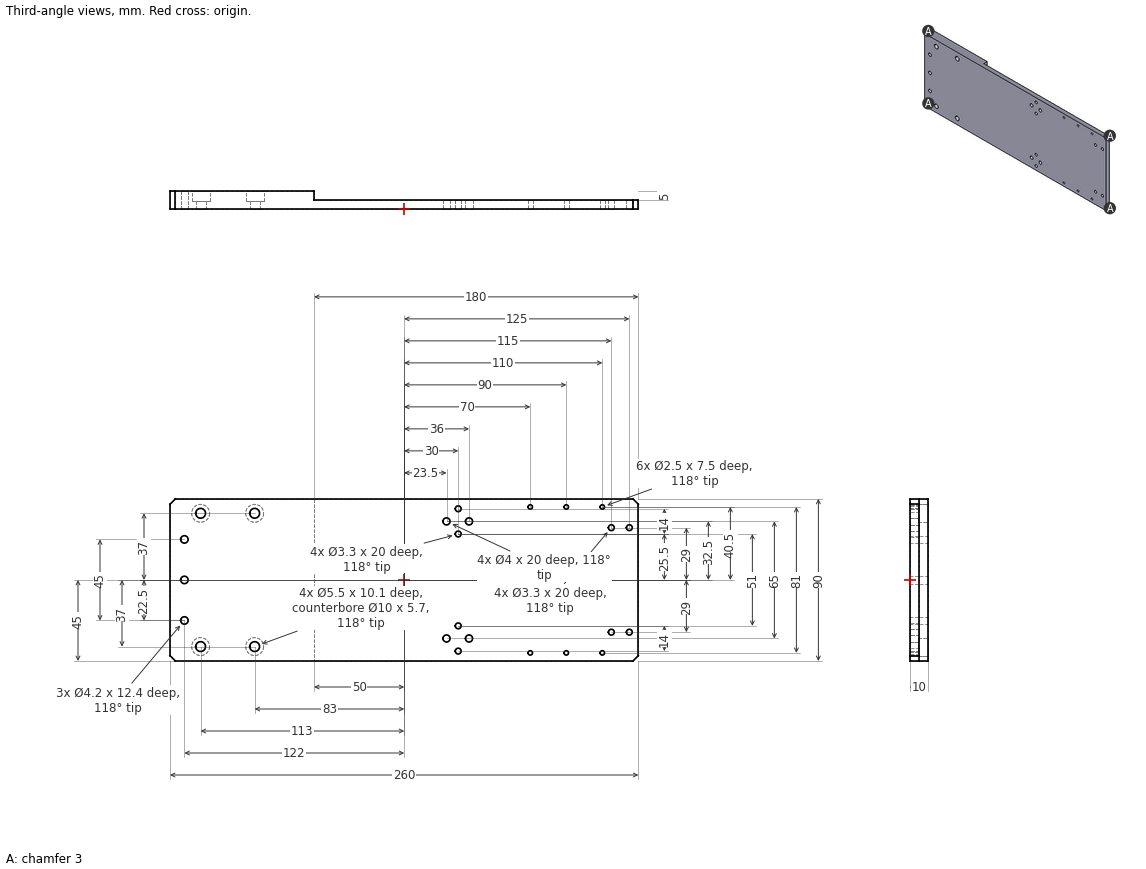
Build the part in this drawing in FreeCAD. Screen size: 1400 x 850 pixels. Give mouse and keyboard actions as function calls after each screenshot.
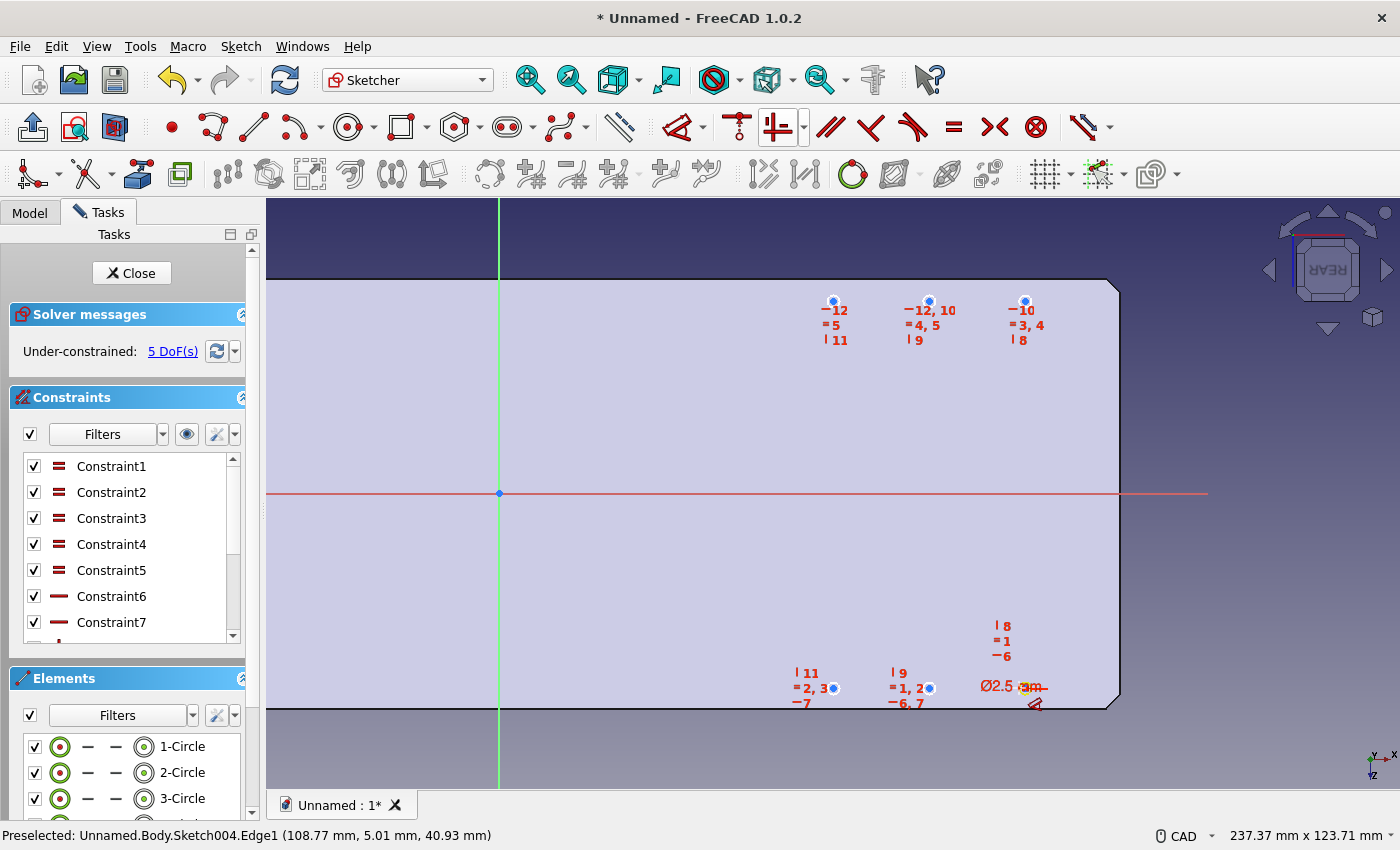
click(929, 689)
click(714, 723)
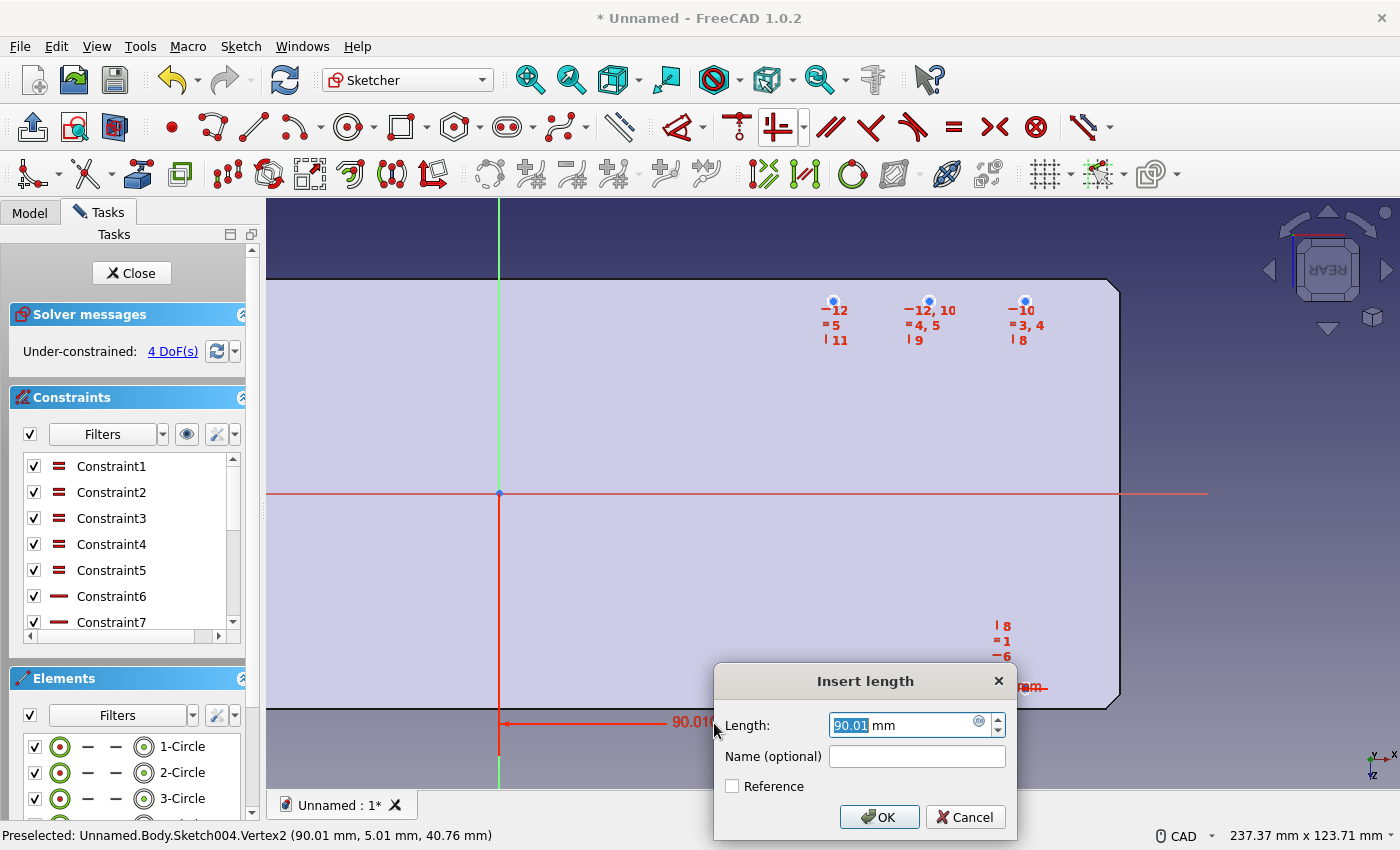
text(90)
key(Return)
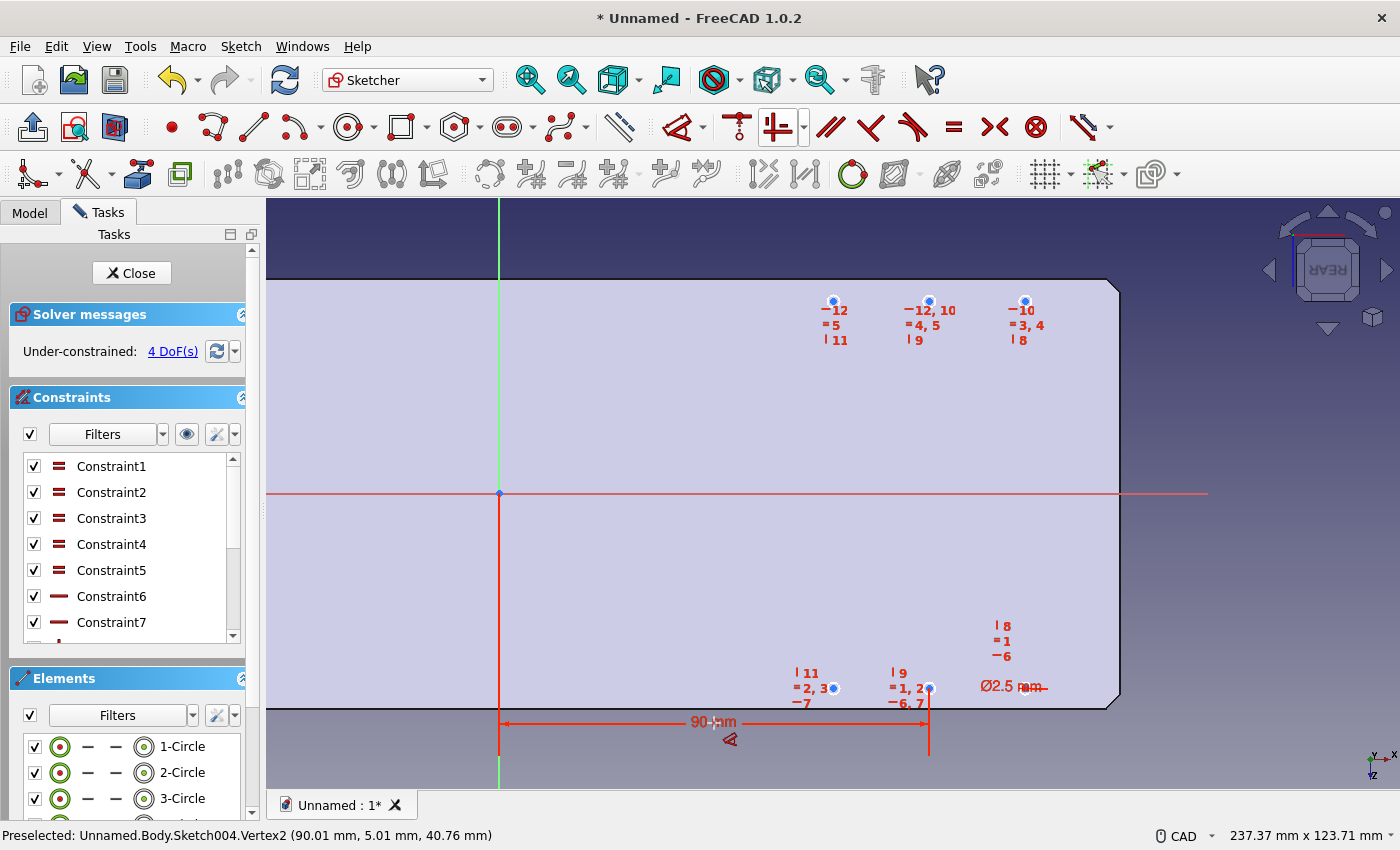
click(834, 689)
click(590, 723)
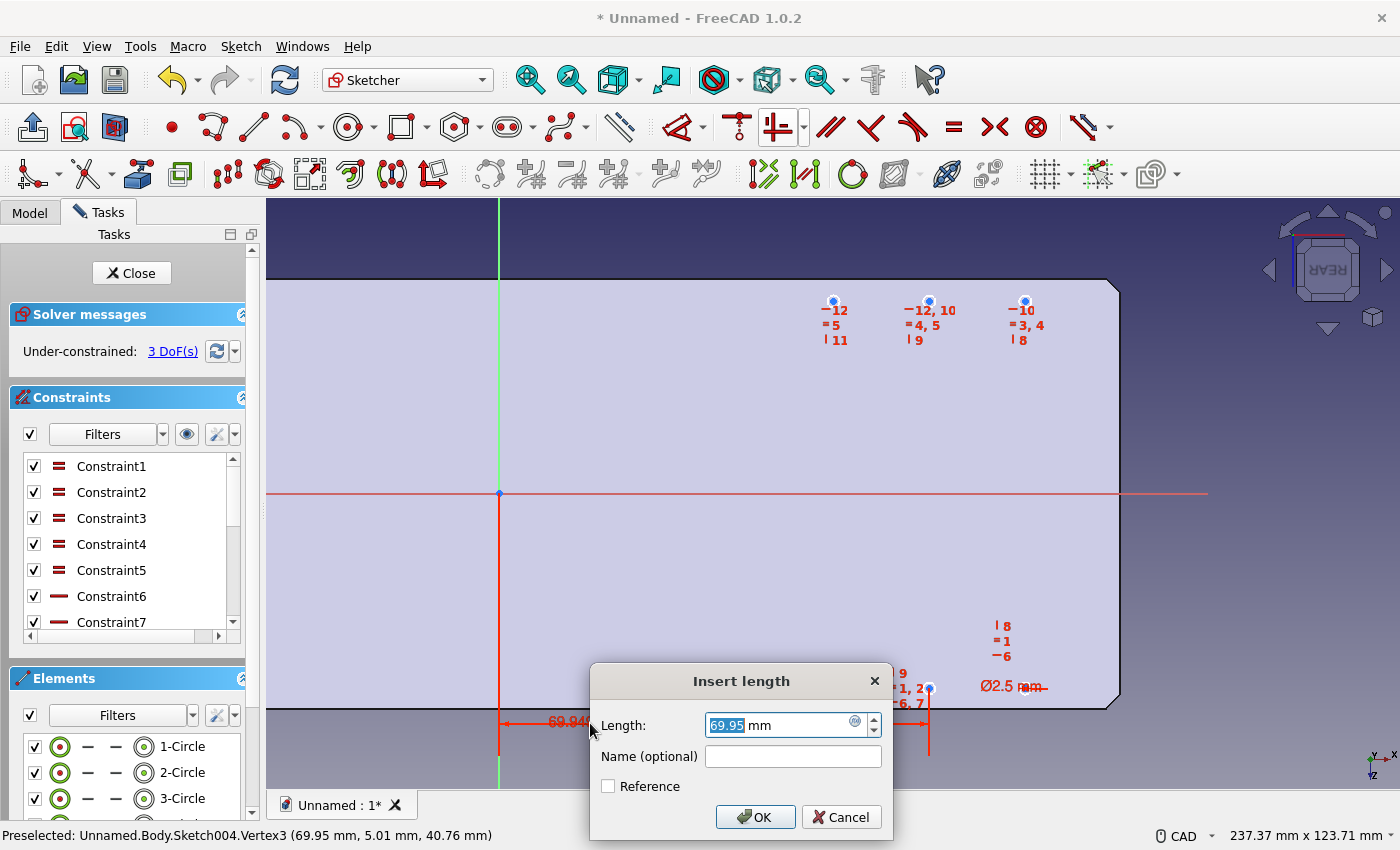
text(70)
key(Return)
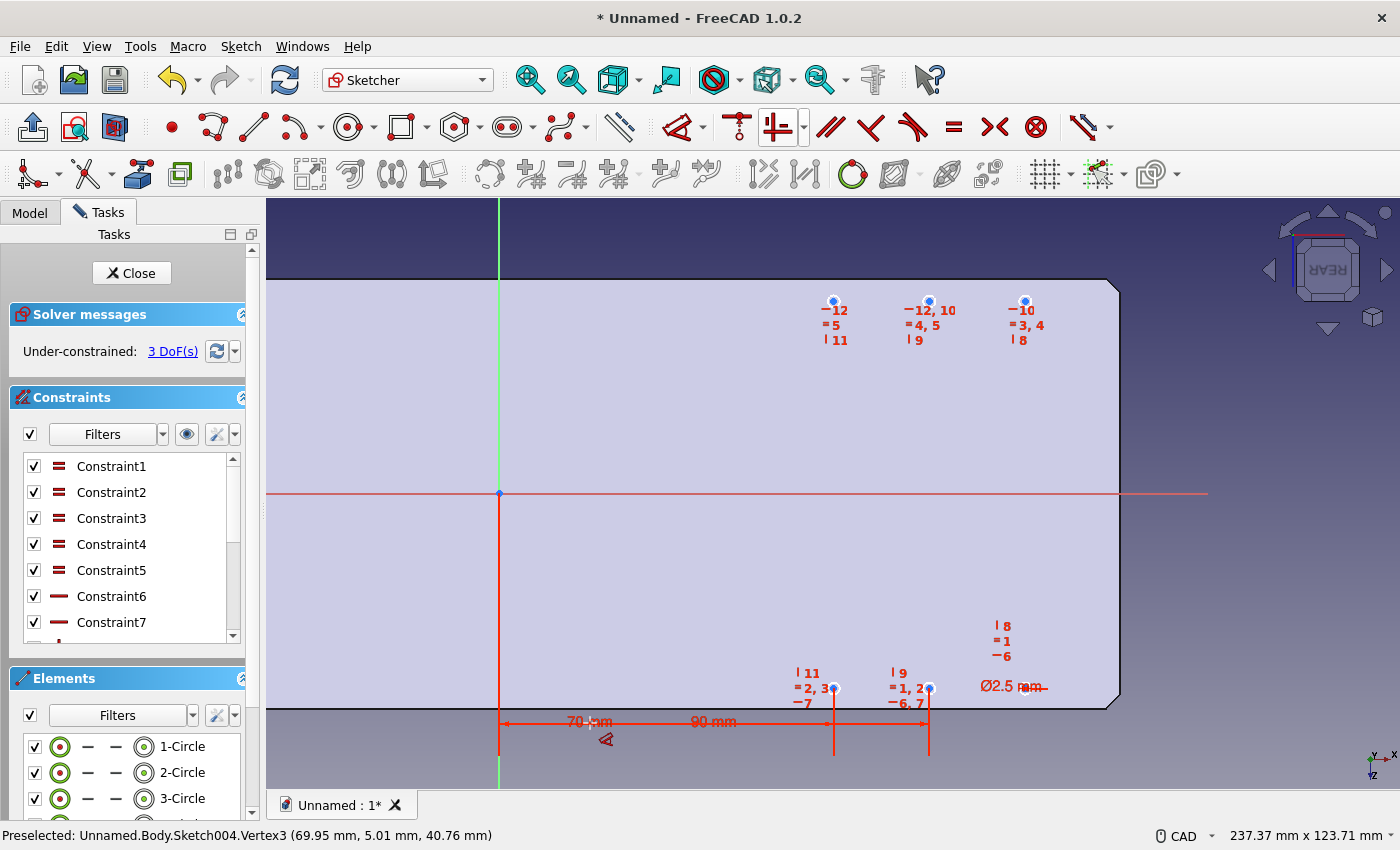
click(1025, 689)
click(883, 723)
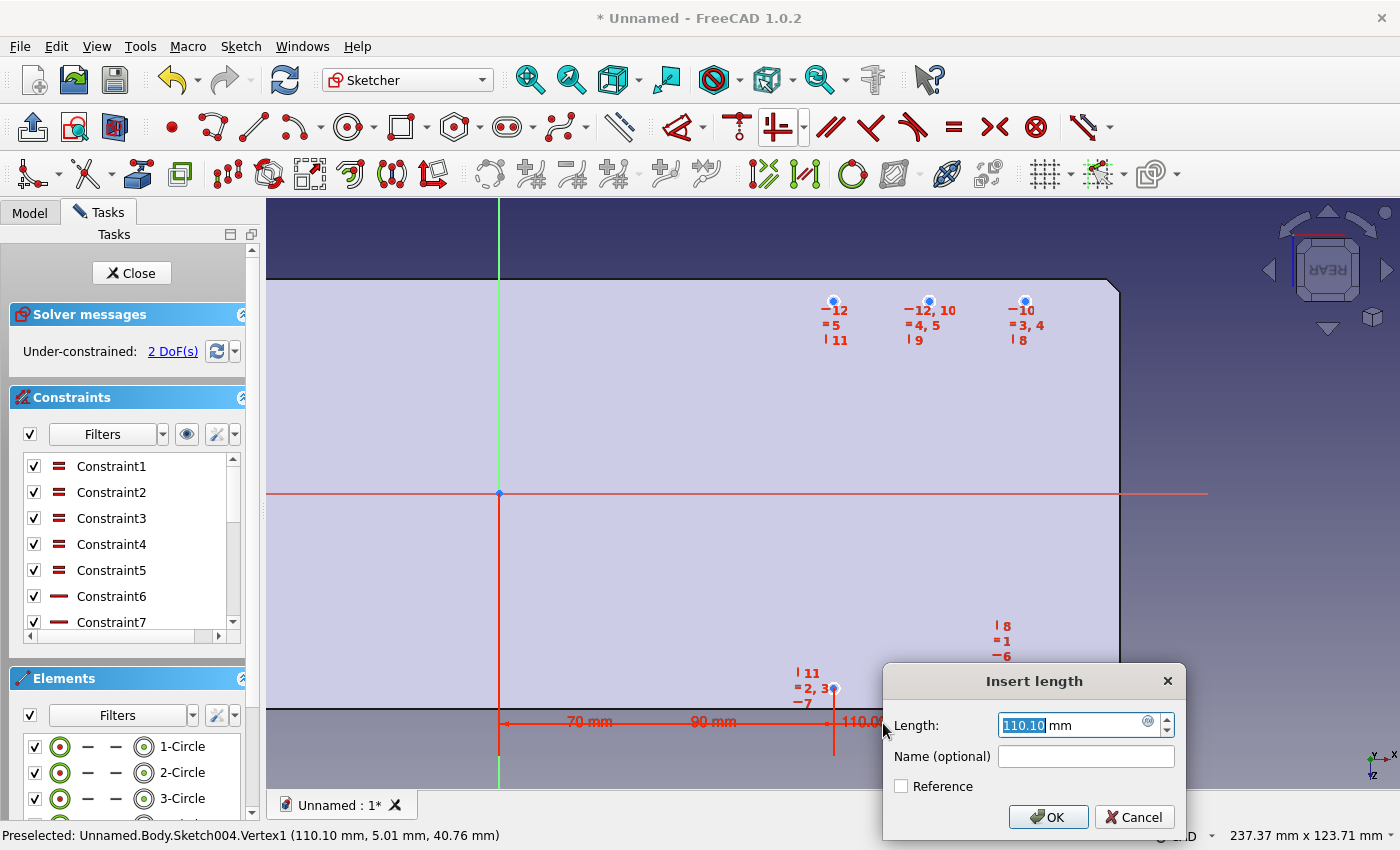
text(110)
key(Return)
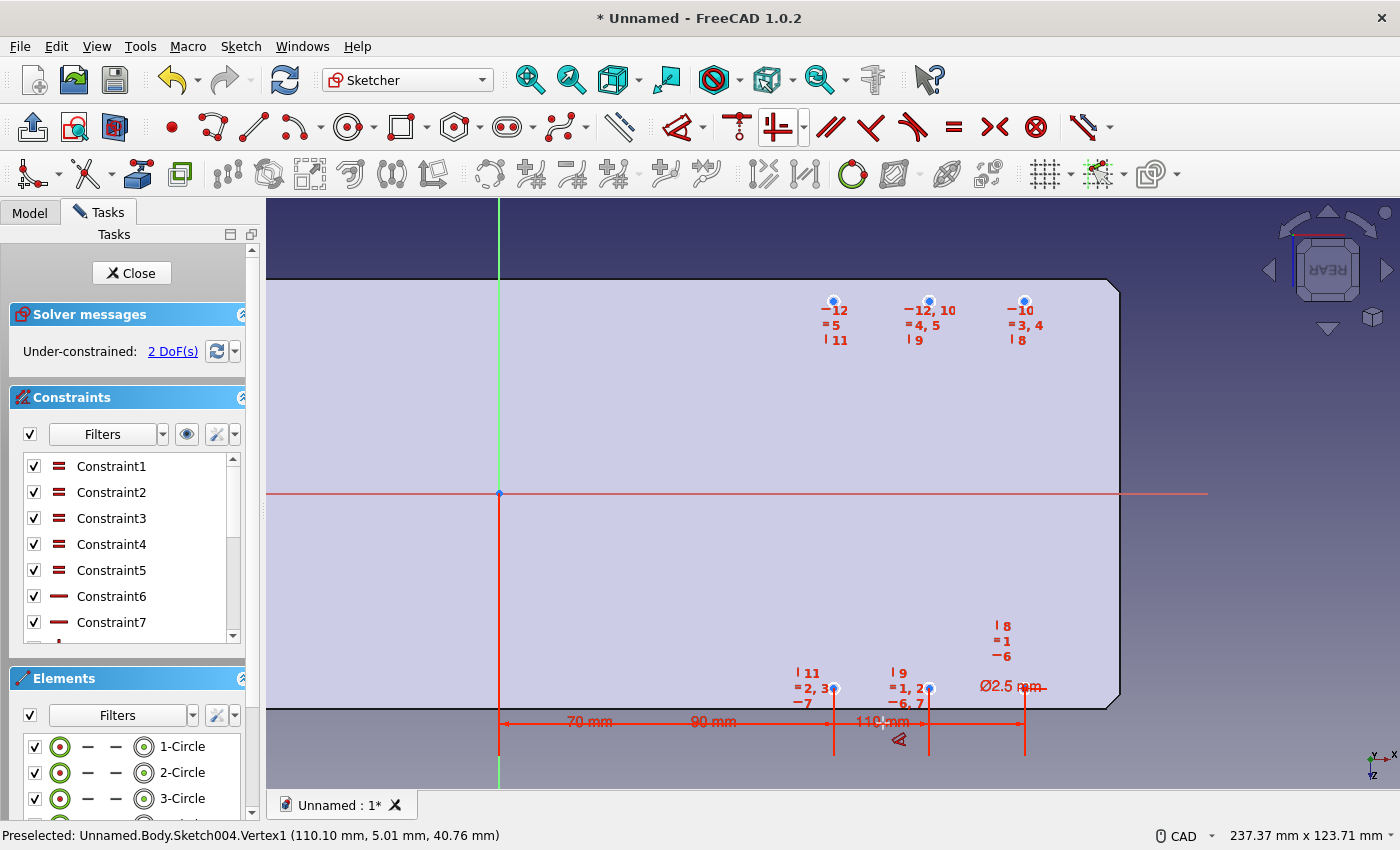
click(1025, 689)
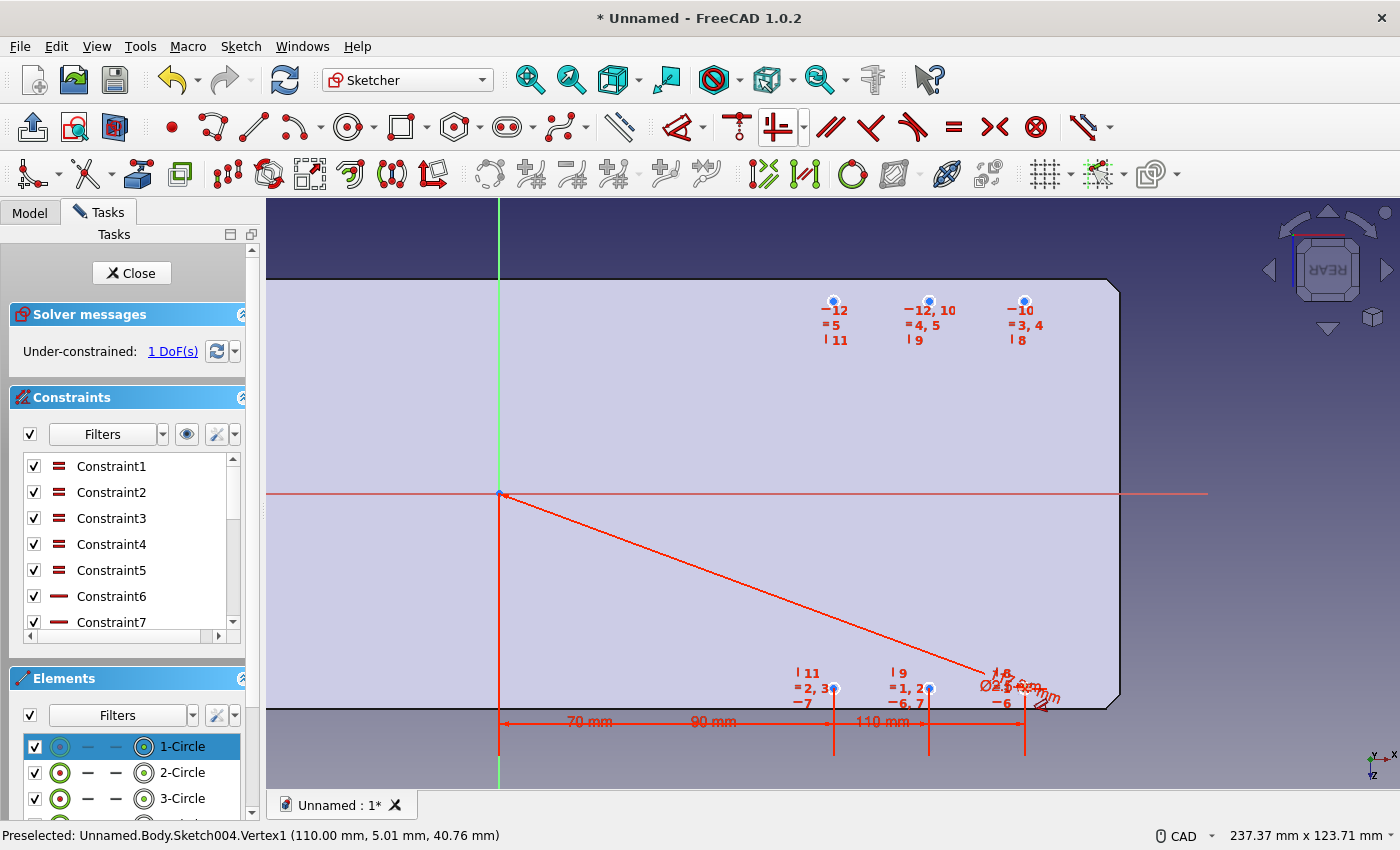
click(1025, 301)
click(1059, 406)